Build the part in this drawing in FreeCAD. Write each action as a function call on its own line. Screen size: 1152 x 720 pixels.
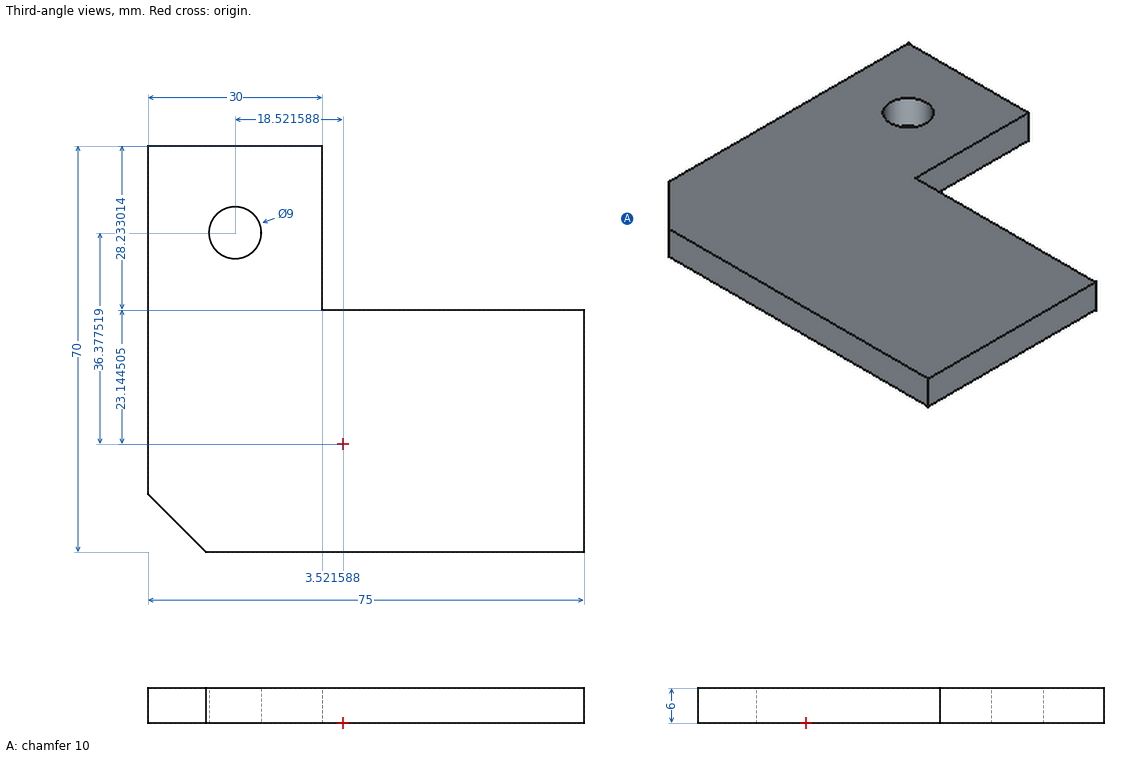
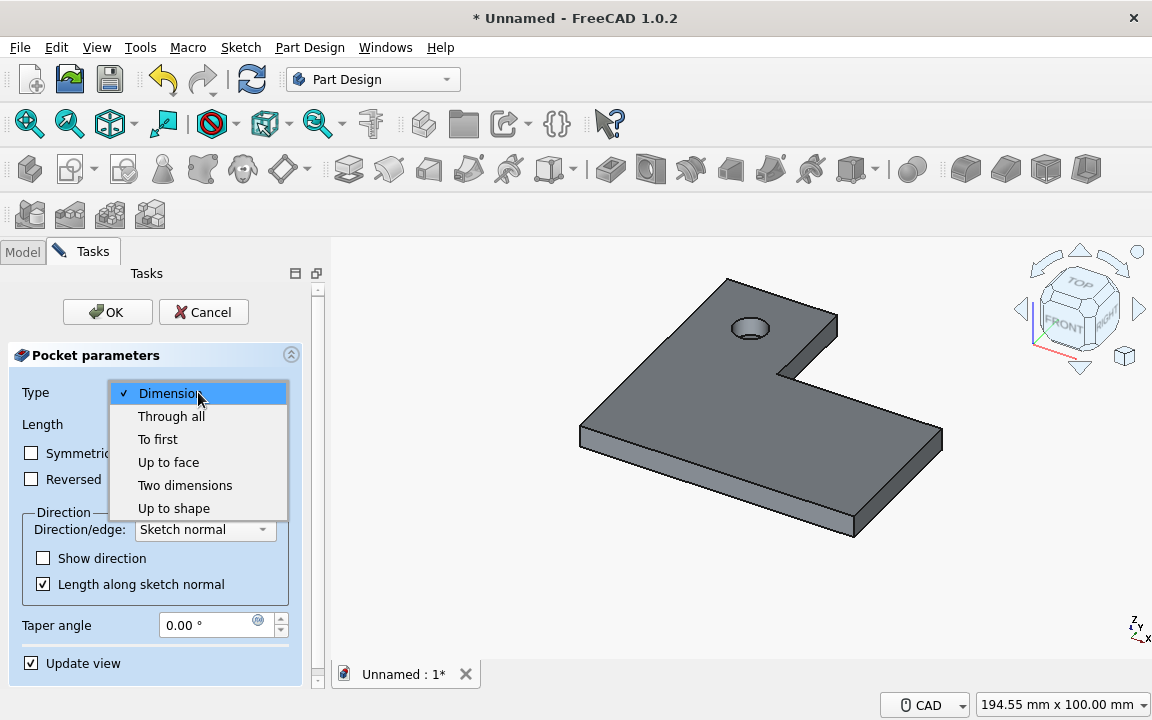
click(198, 440)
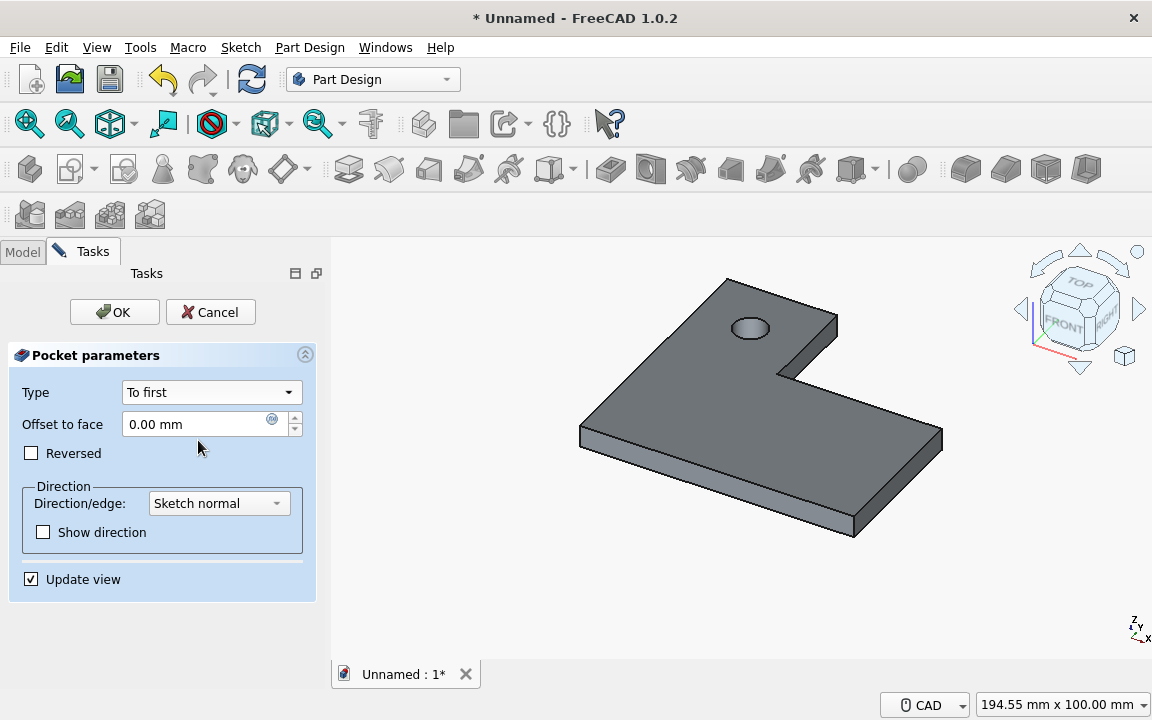
click(115, 312)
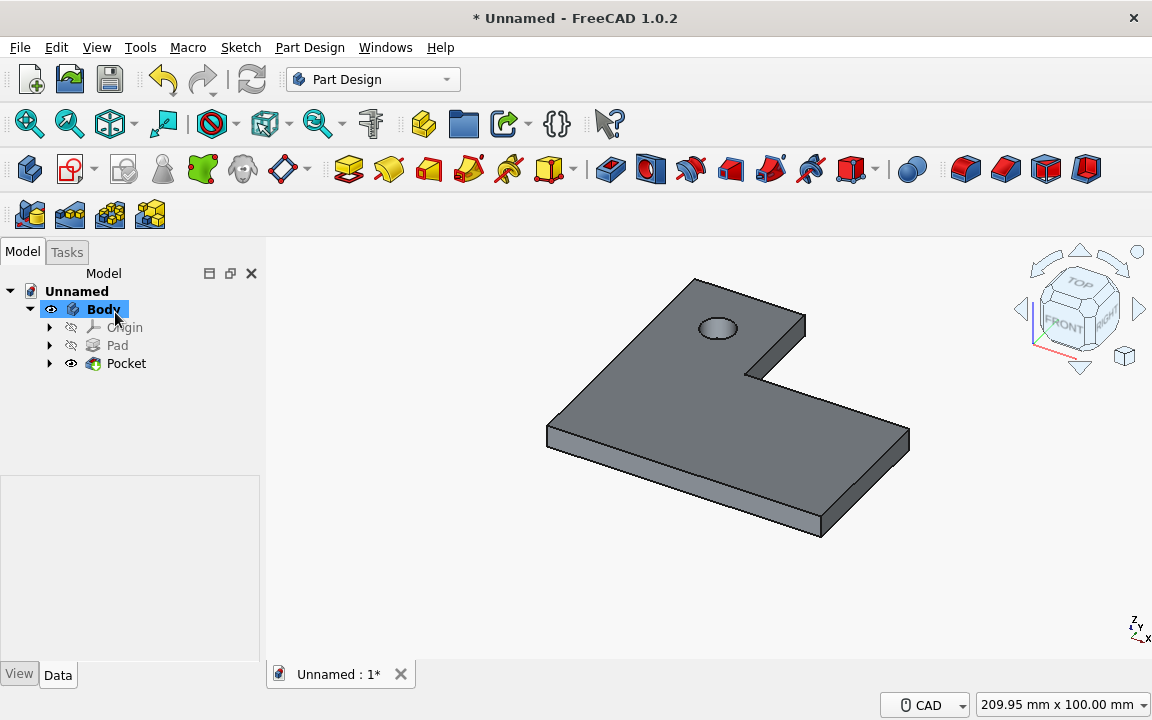
key(0)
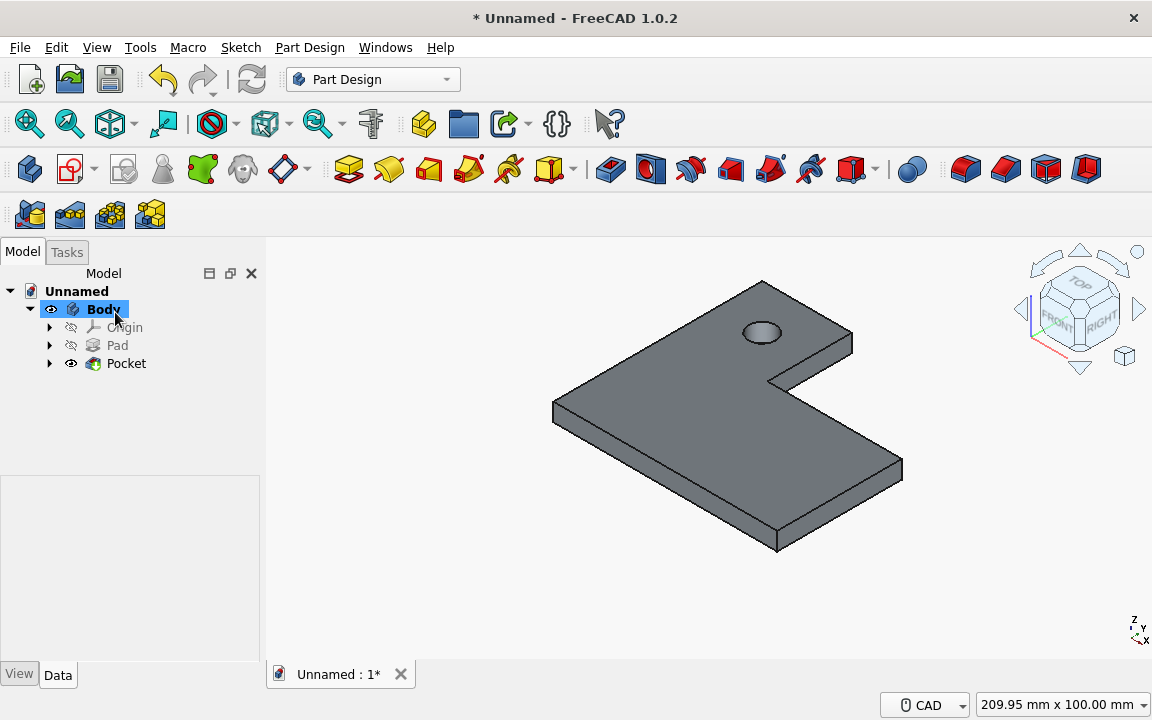
key(2)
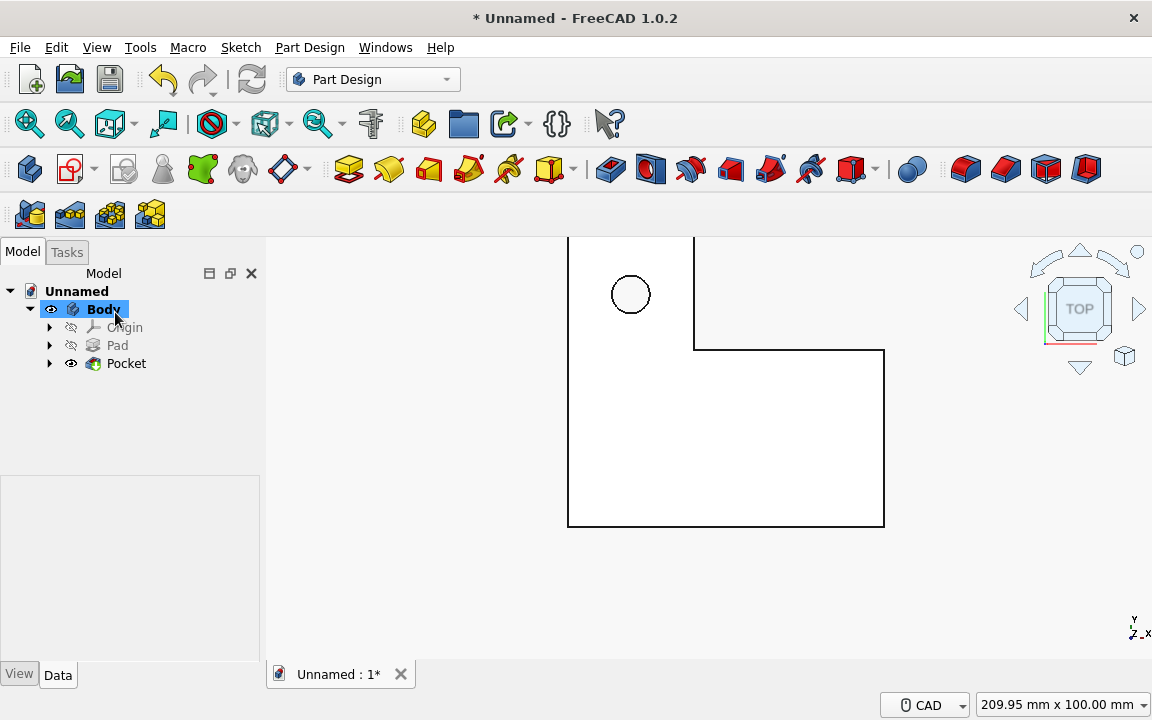
click(30, 124)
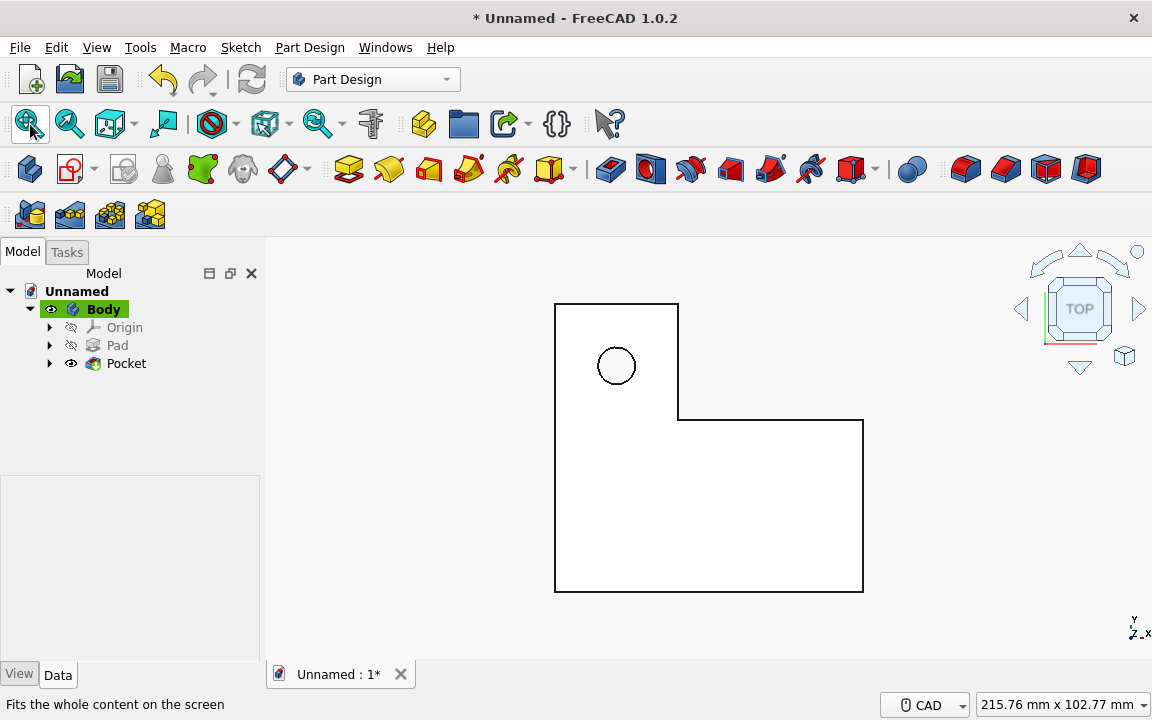
key(1)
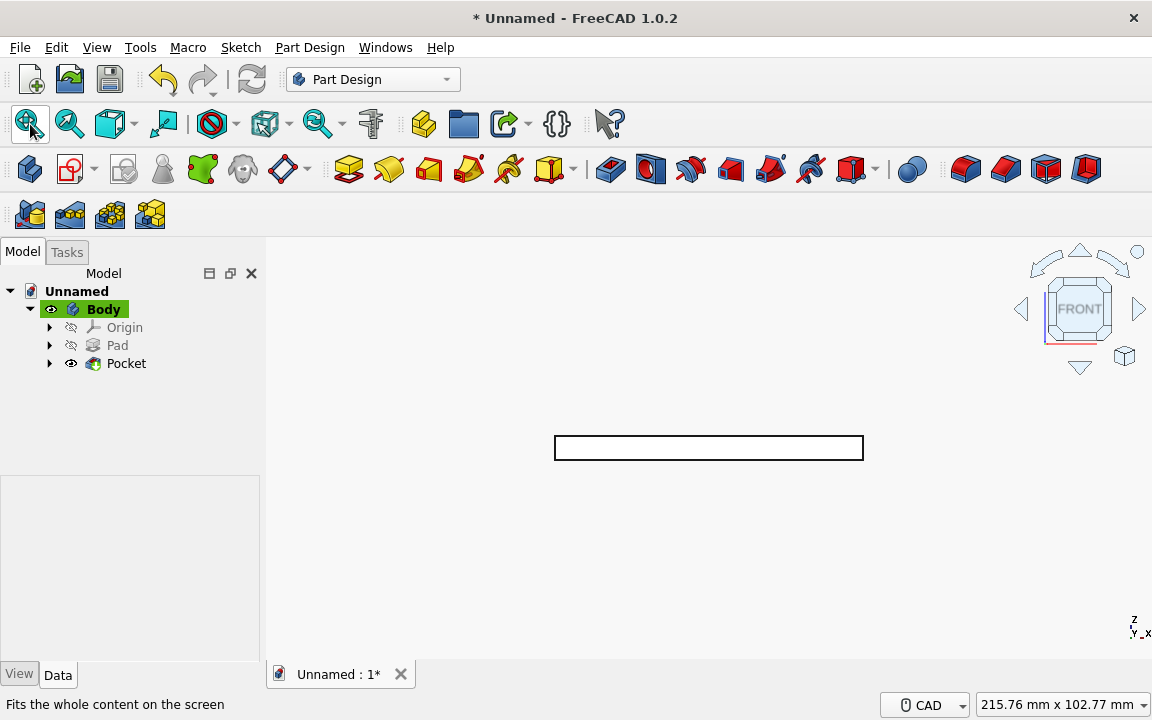
click(30, 124)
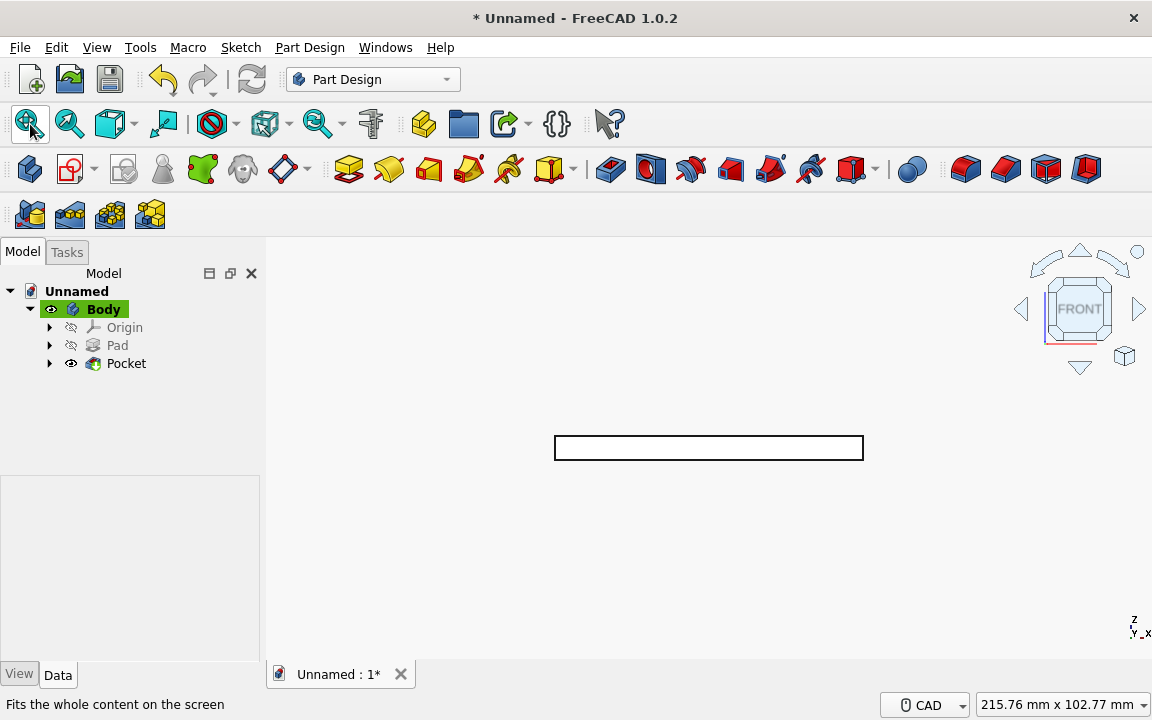
click(555, 447)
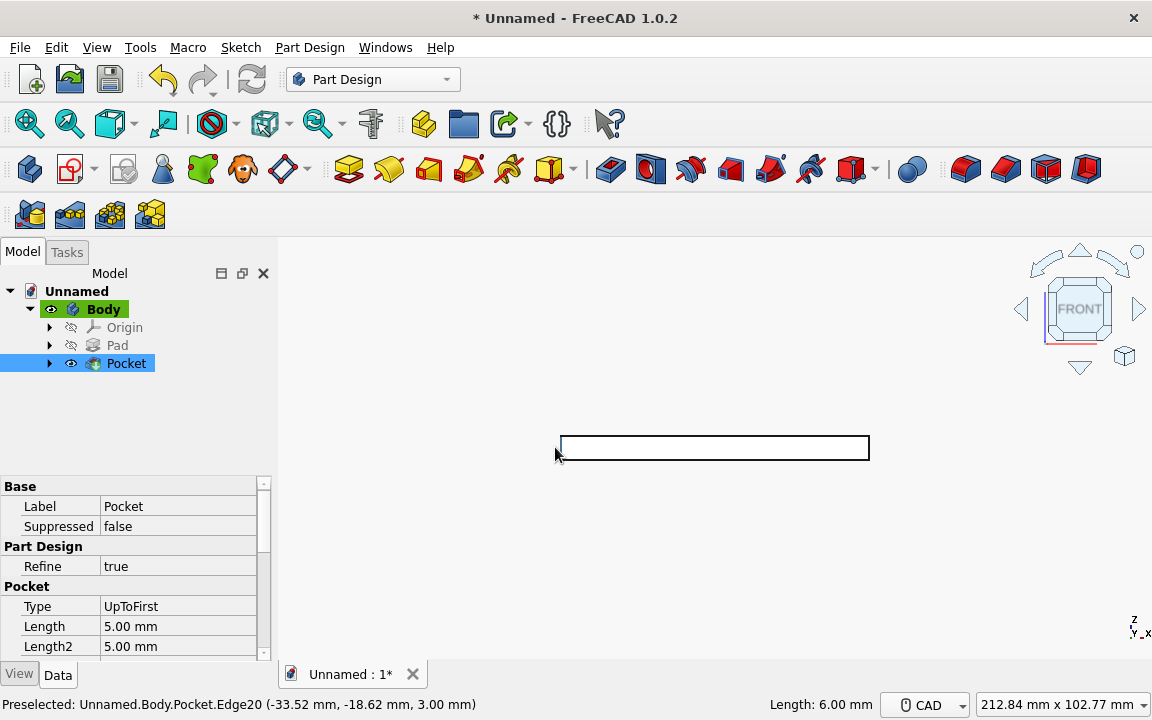
click(1006, 170)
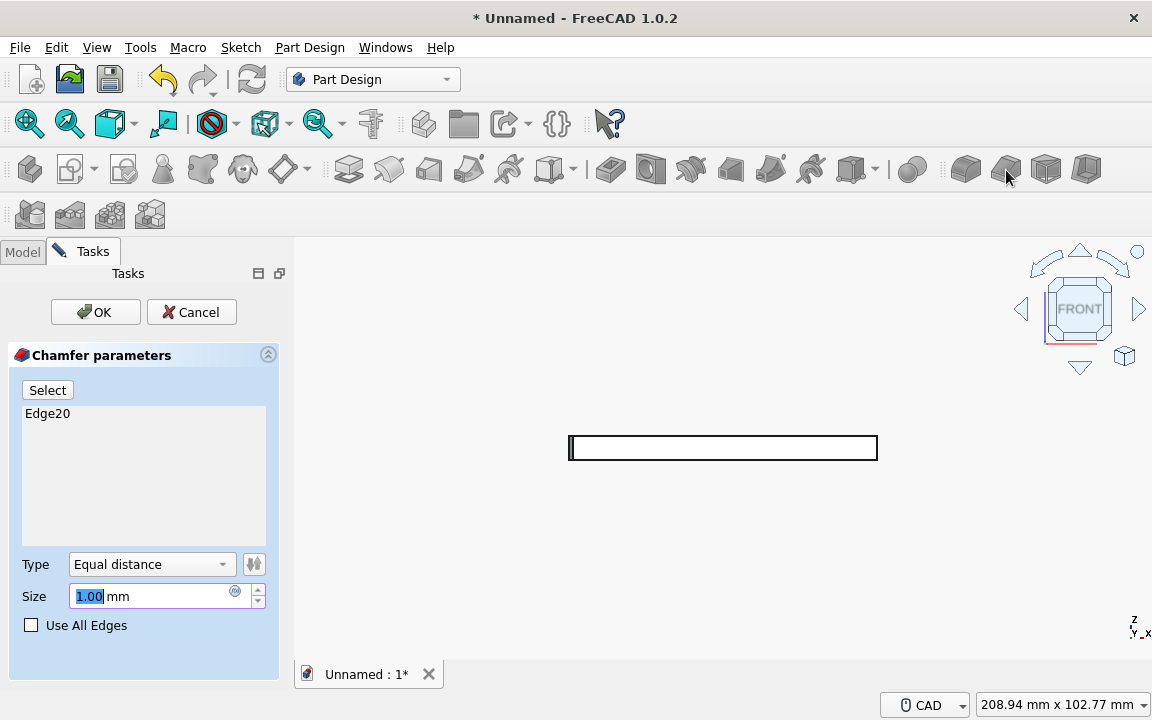
text(10)
key(Tab)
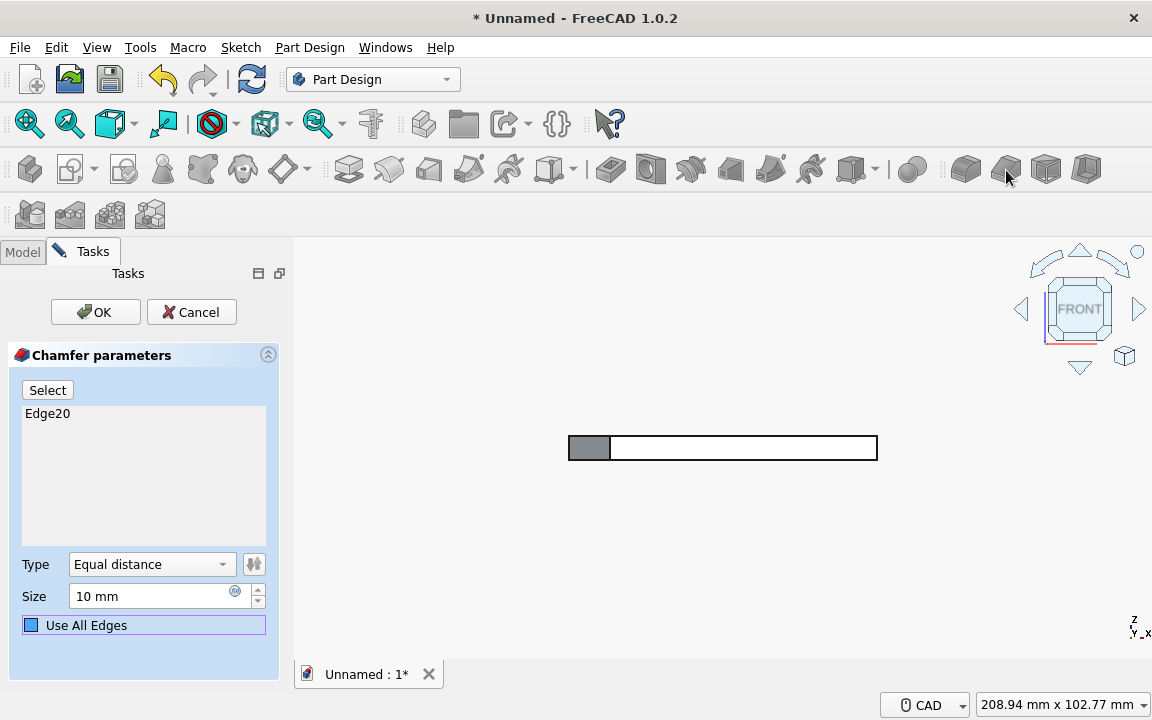
click(96, 312)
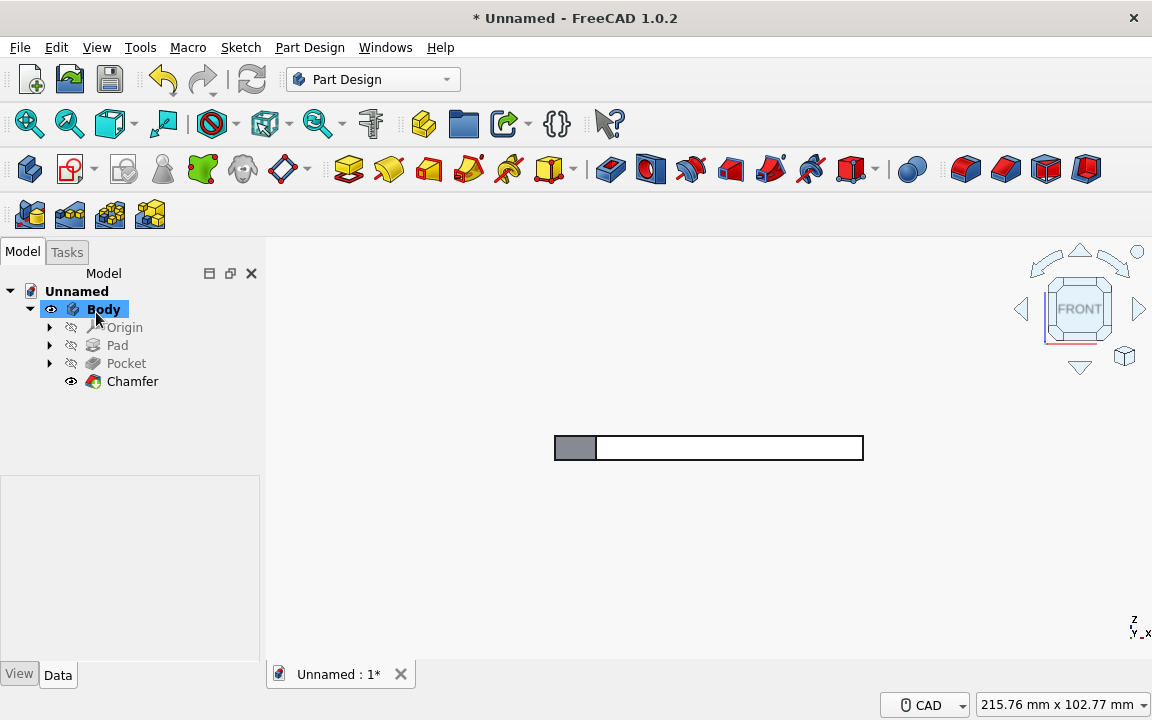
key(0)